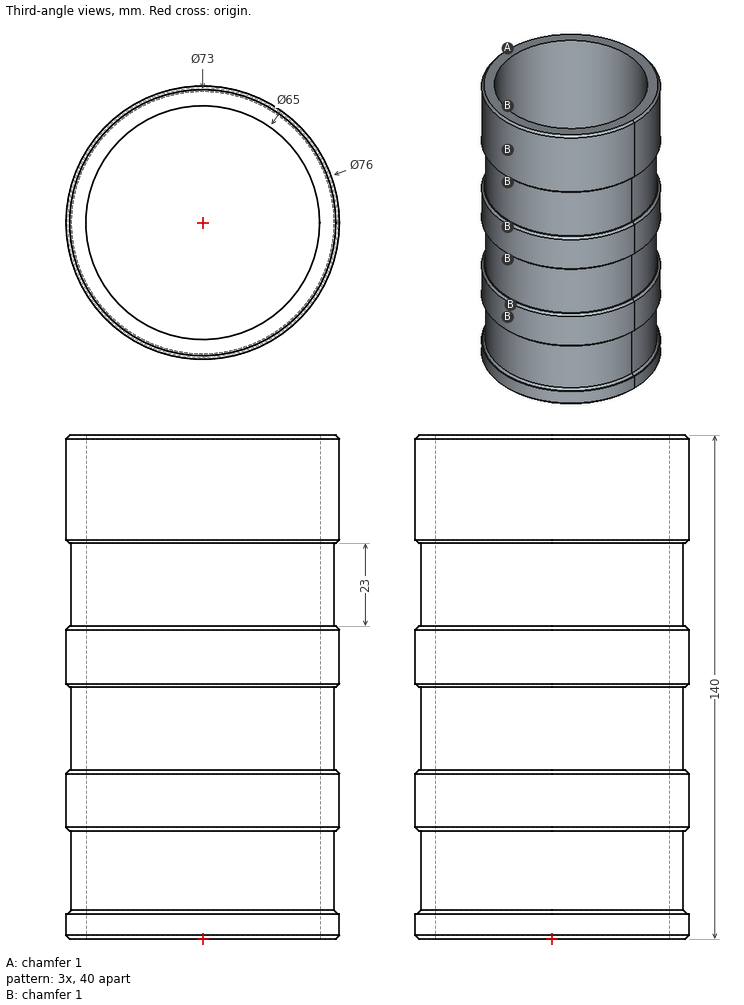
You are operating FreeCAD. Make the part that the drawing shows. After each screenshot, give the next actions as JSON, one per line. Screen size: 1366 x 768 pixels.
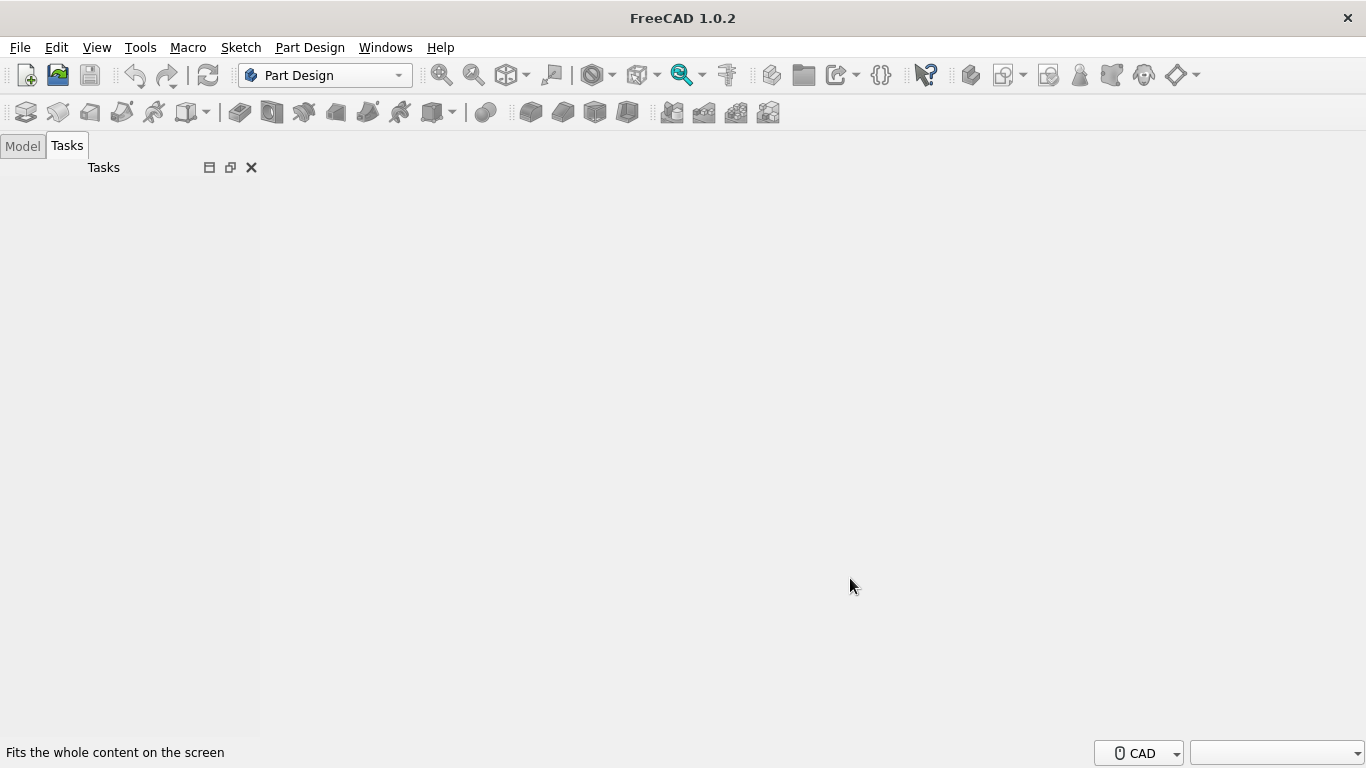
{"action": "left_click", "coordinate": [26, 76]}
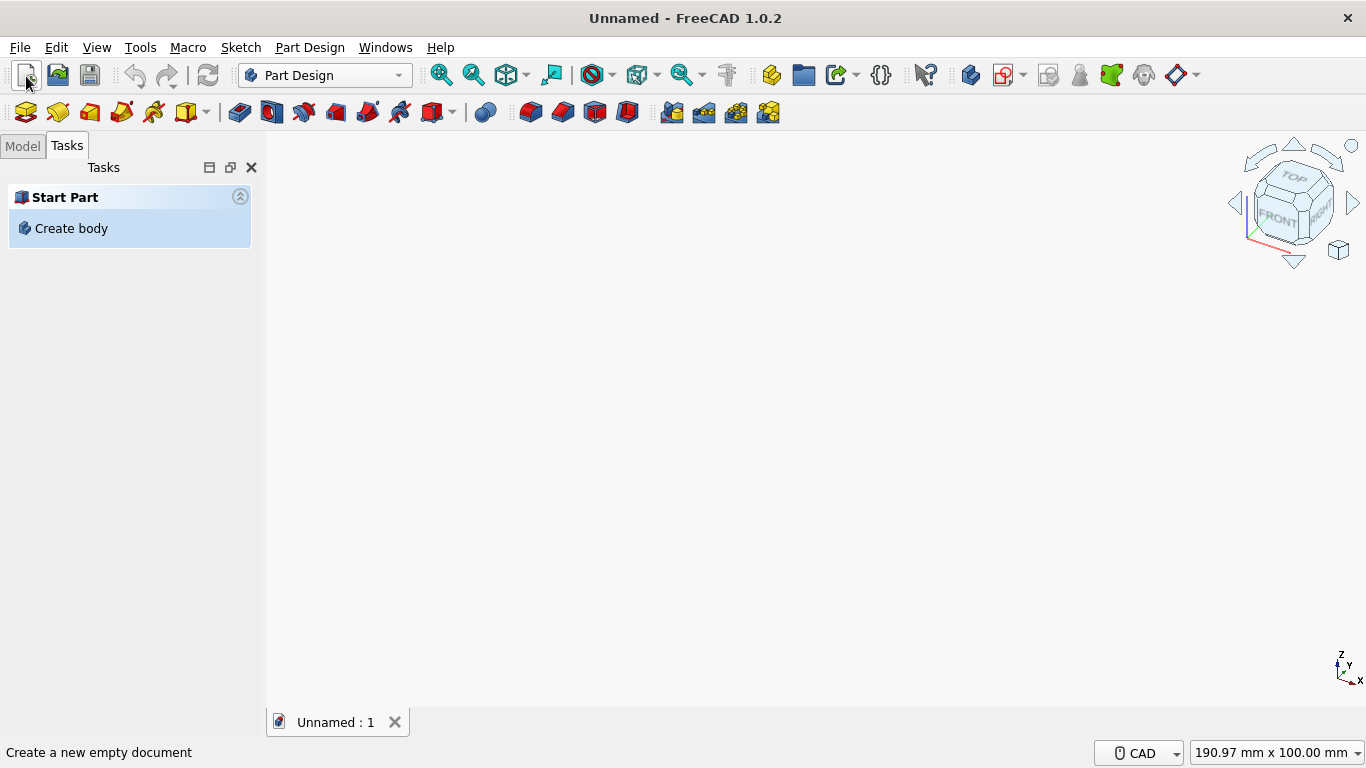
{"action": "left_click", "coordinate": [1004, 76]}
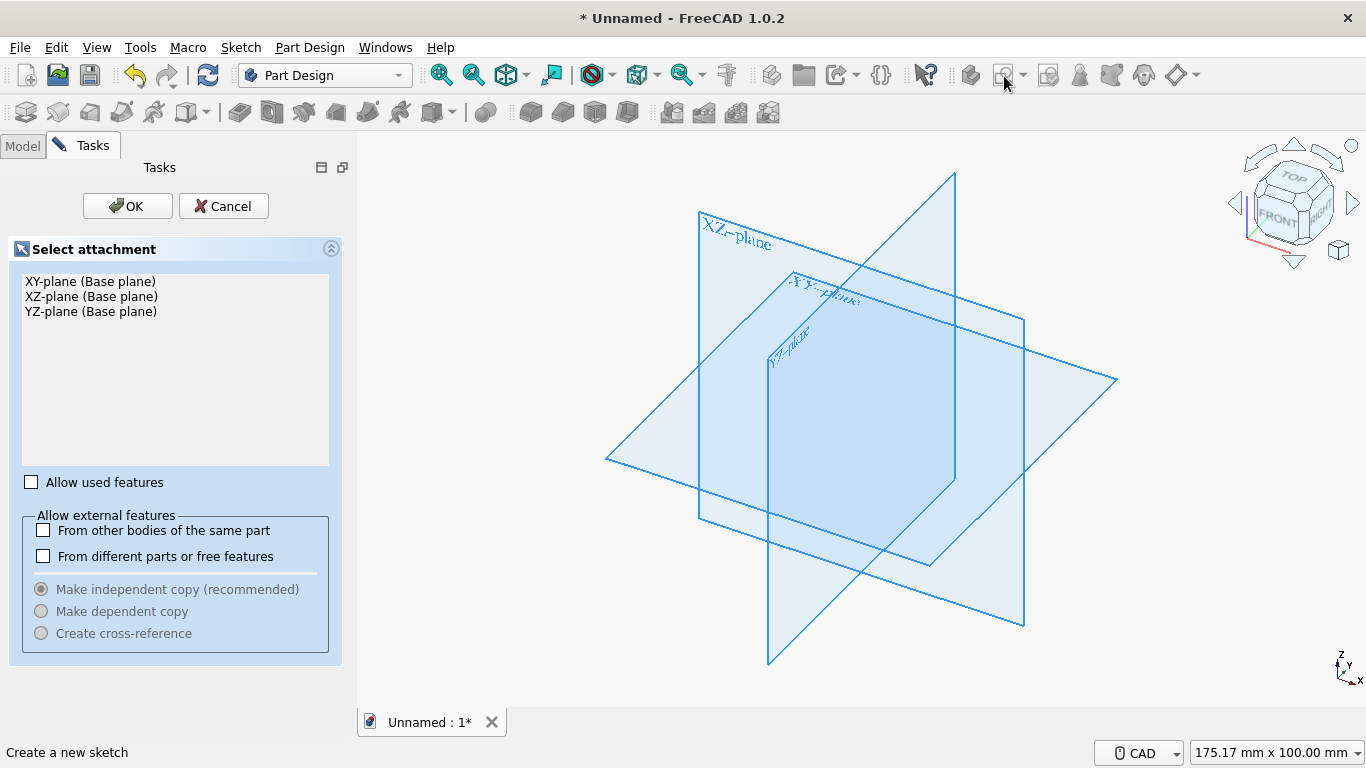
{"action": "left_click", "coordinate": [82, 282]}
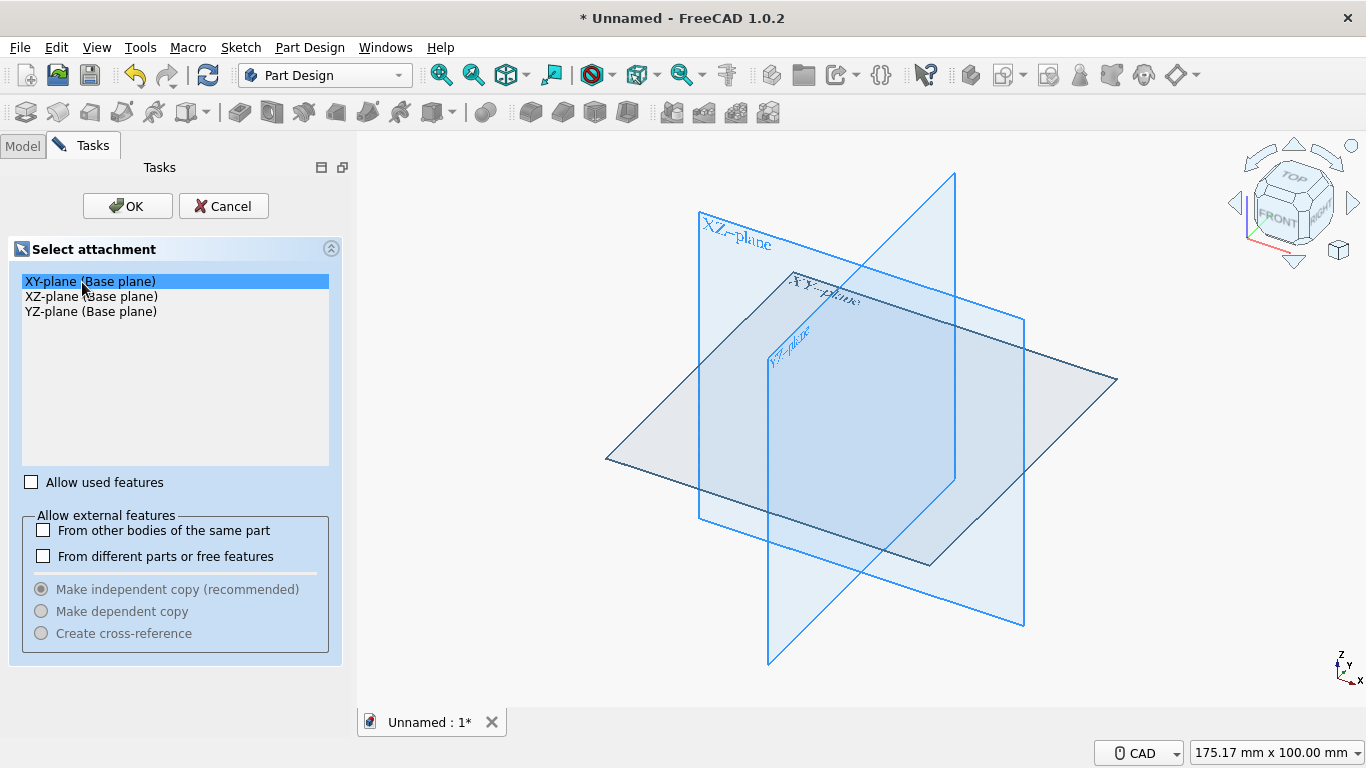
{"action": "left_click", "coordinate": [128, 206]}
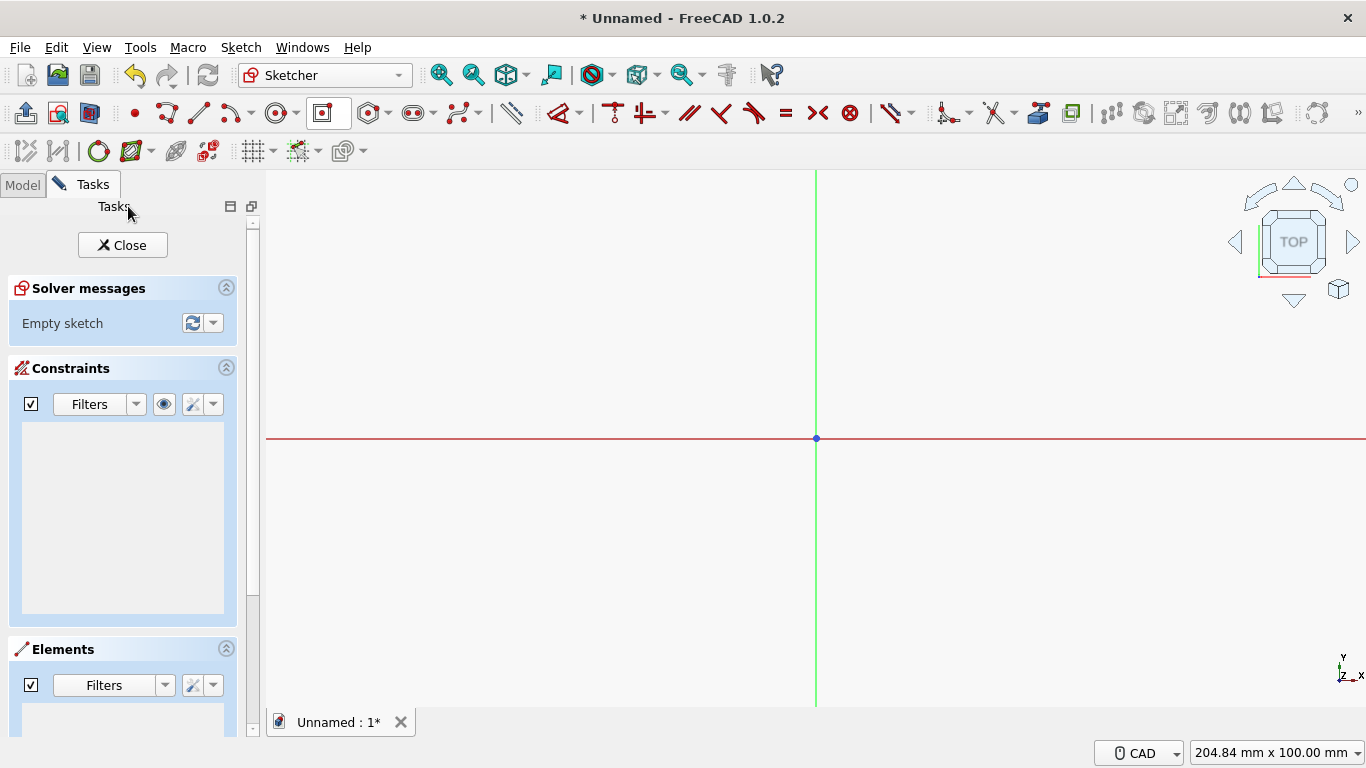
{"action": "left_click", "coordinate": [276, 114]}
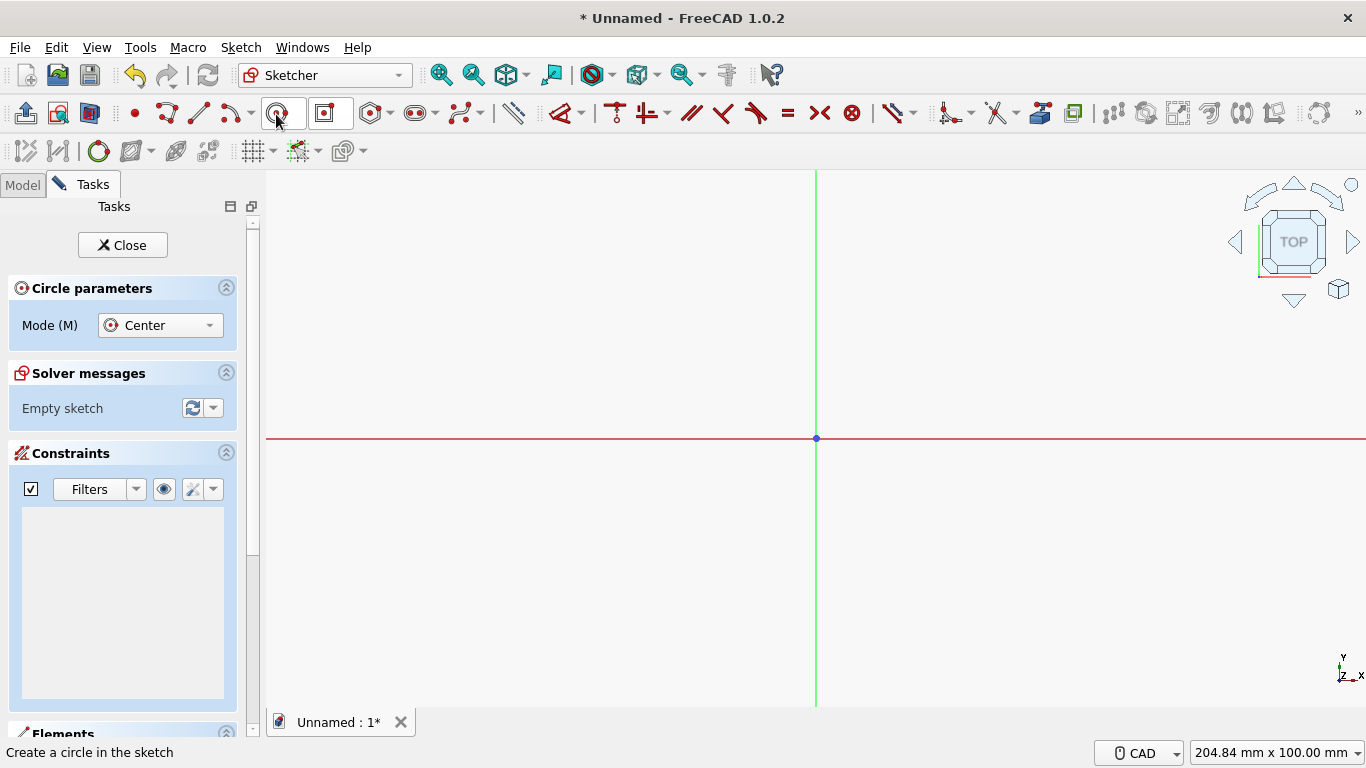
{"action": "left_click", "coordinate": [816, 438]}
{"action": "left_click", "coordinate": [960, 294]}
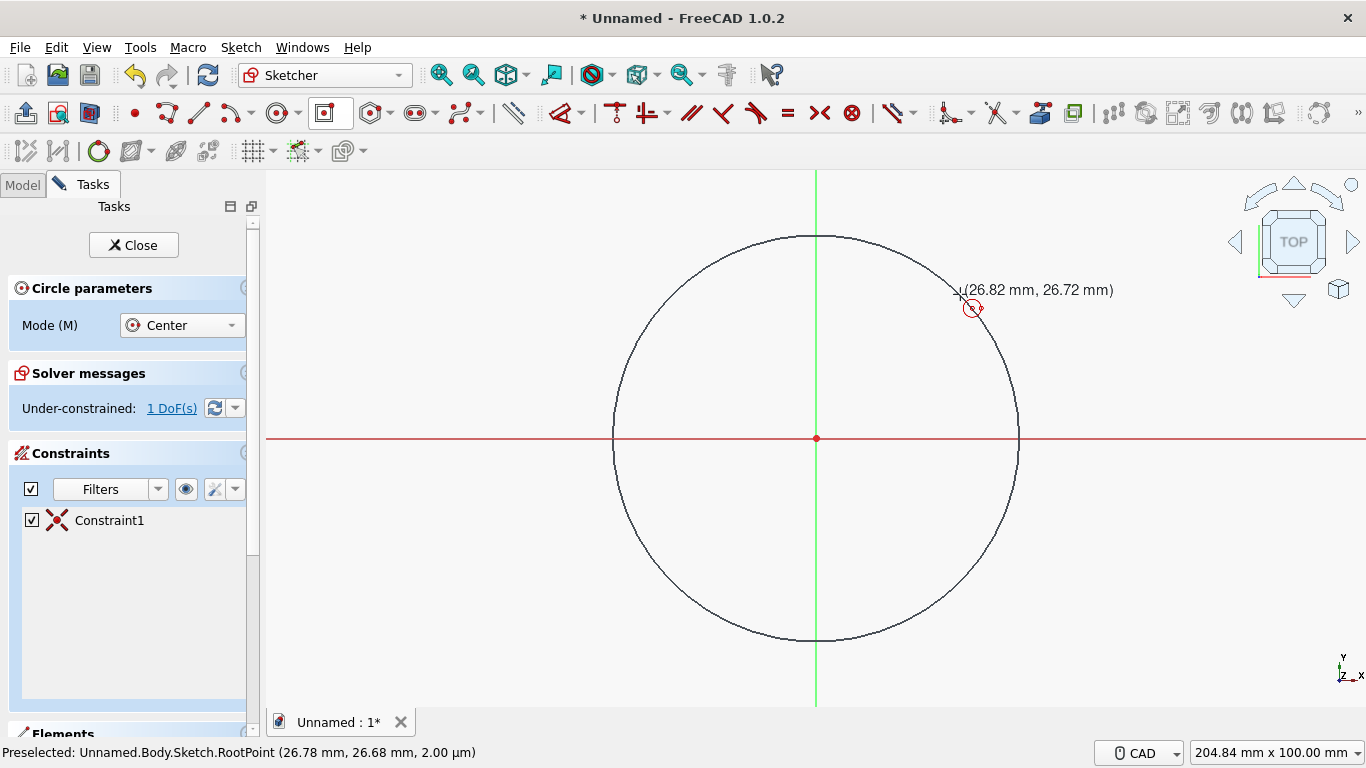
{"action": "left_click", "coordinate": [816, 438]}
{"action": "left_click", "coordinate": [939, 315]}
{"action": "key", "text": "Escape"}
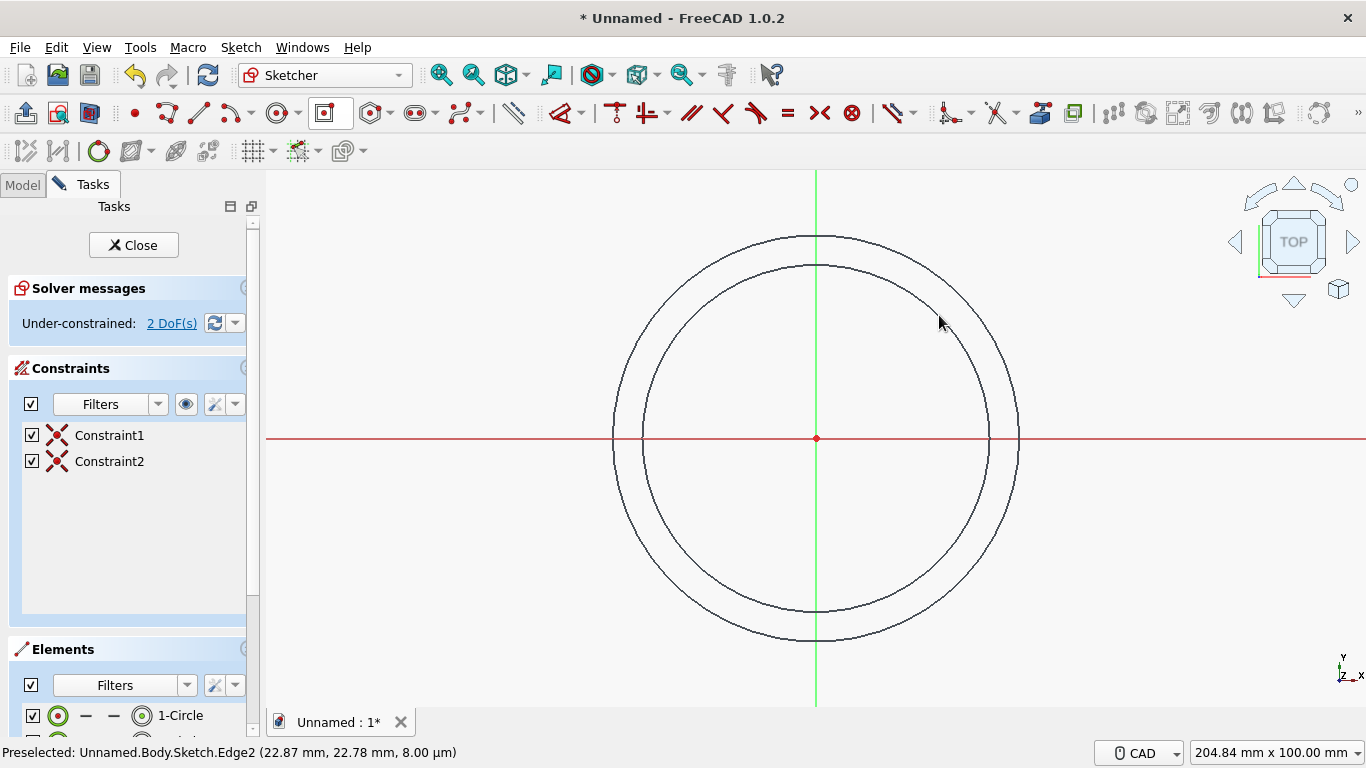
{"action": "left_click", "coordinate": [959, 294]}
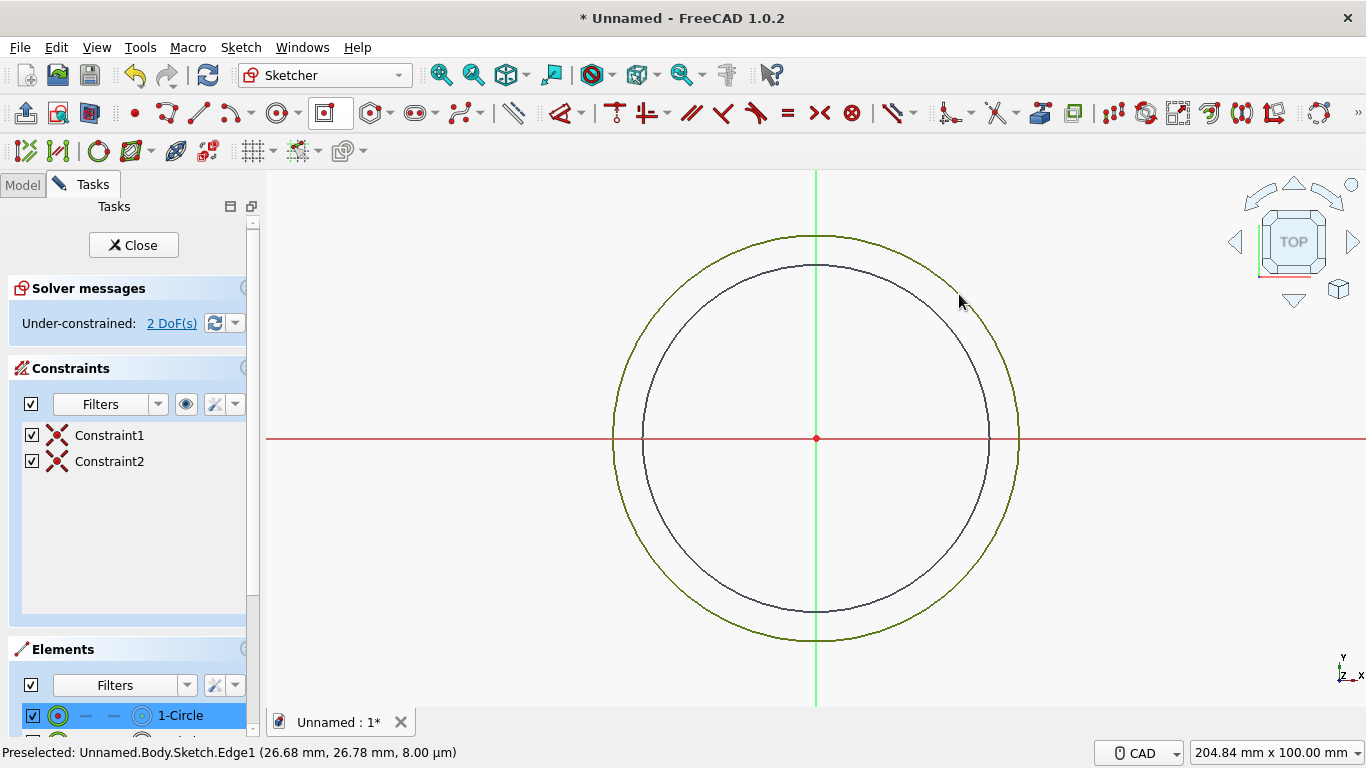
{"action": "key", "text": "k o"}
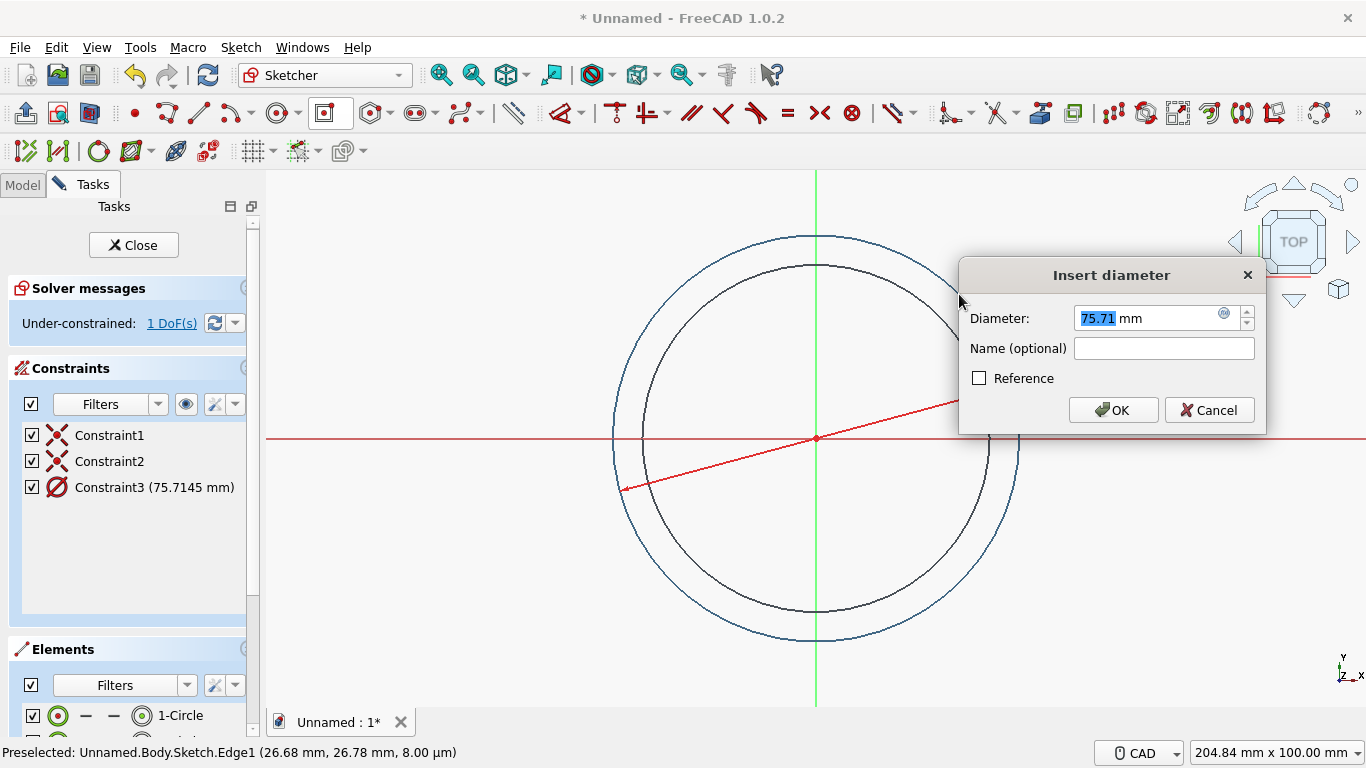
{"action": "type", "text": "76"}
{"action": "key", "text": "Return"}